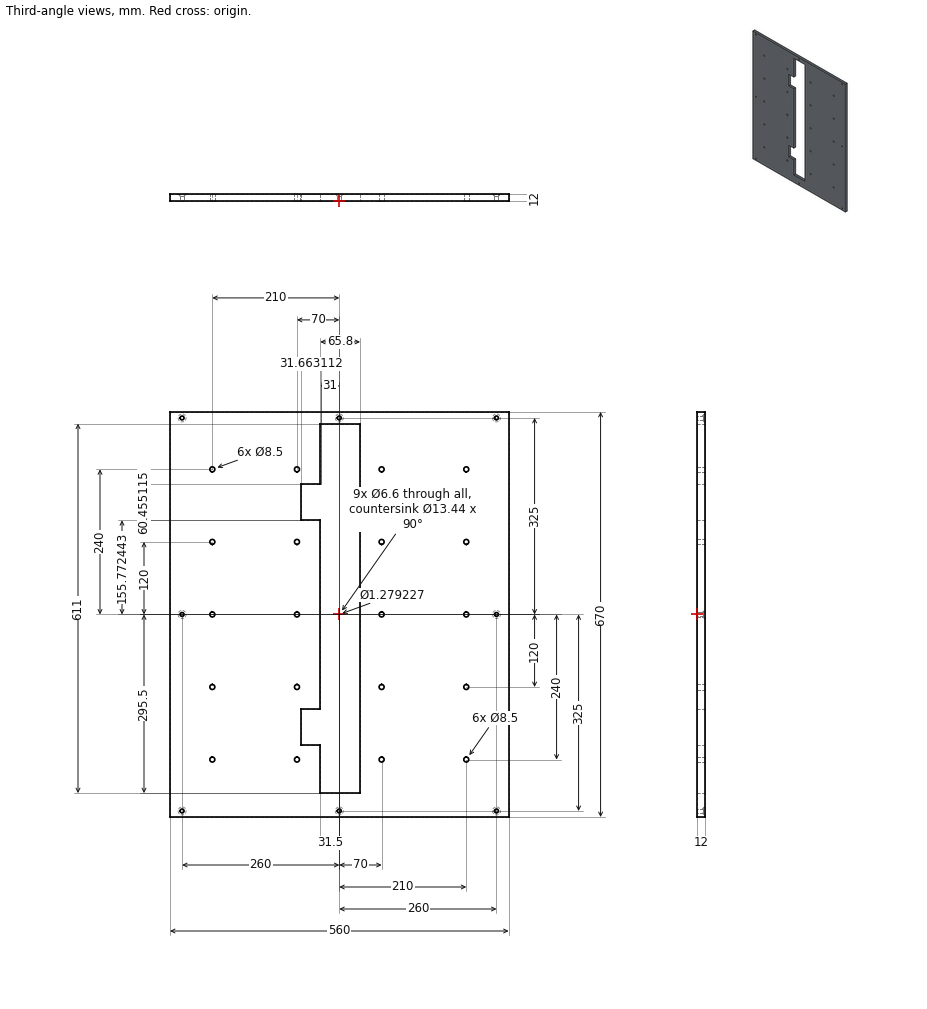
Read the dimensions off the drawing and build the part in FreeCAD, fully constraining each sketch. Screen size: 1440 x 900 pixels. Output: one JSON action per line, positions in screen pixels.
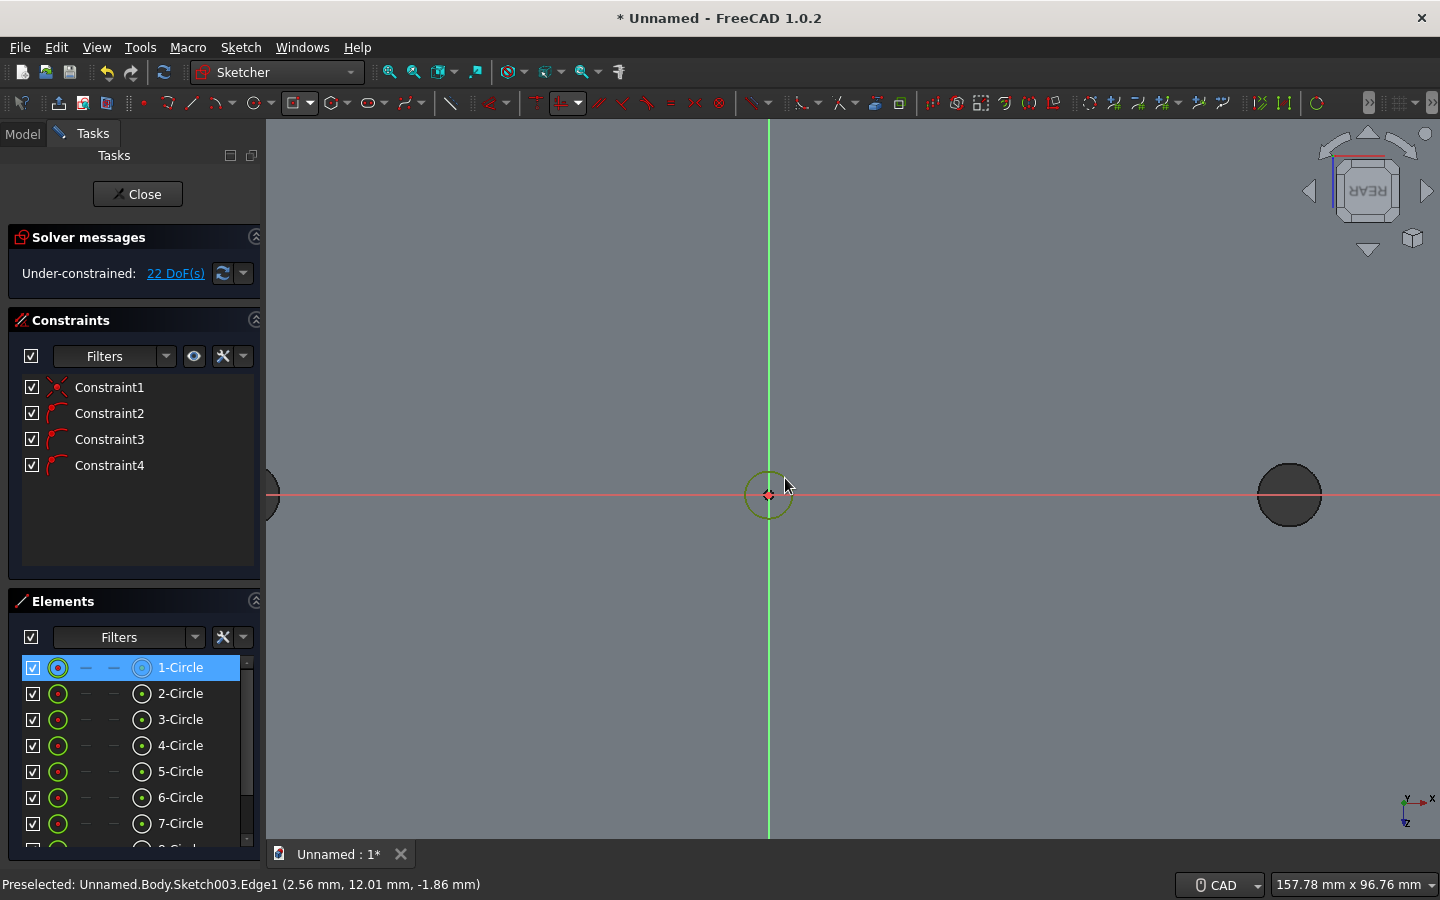
{"action": "scroll", "coordinate": [786, 477], "scroll_direction": "down", "scroll_amount": 12}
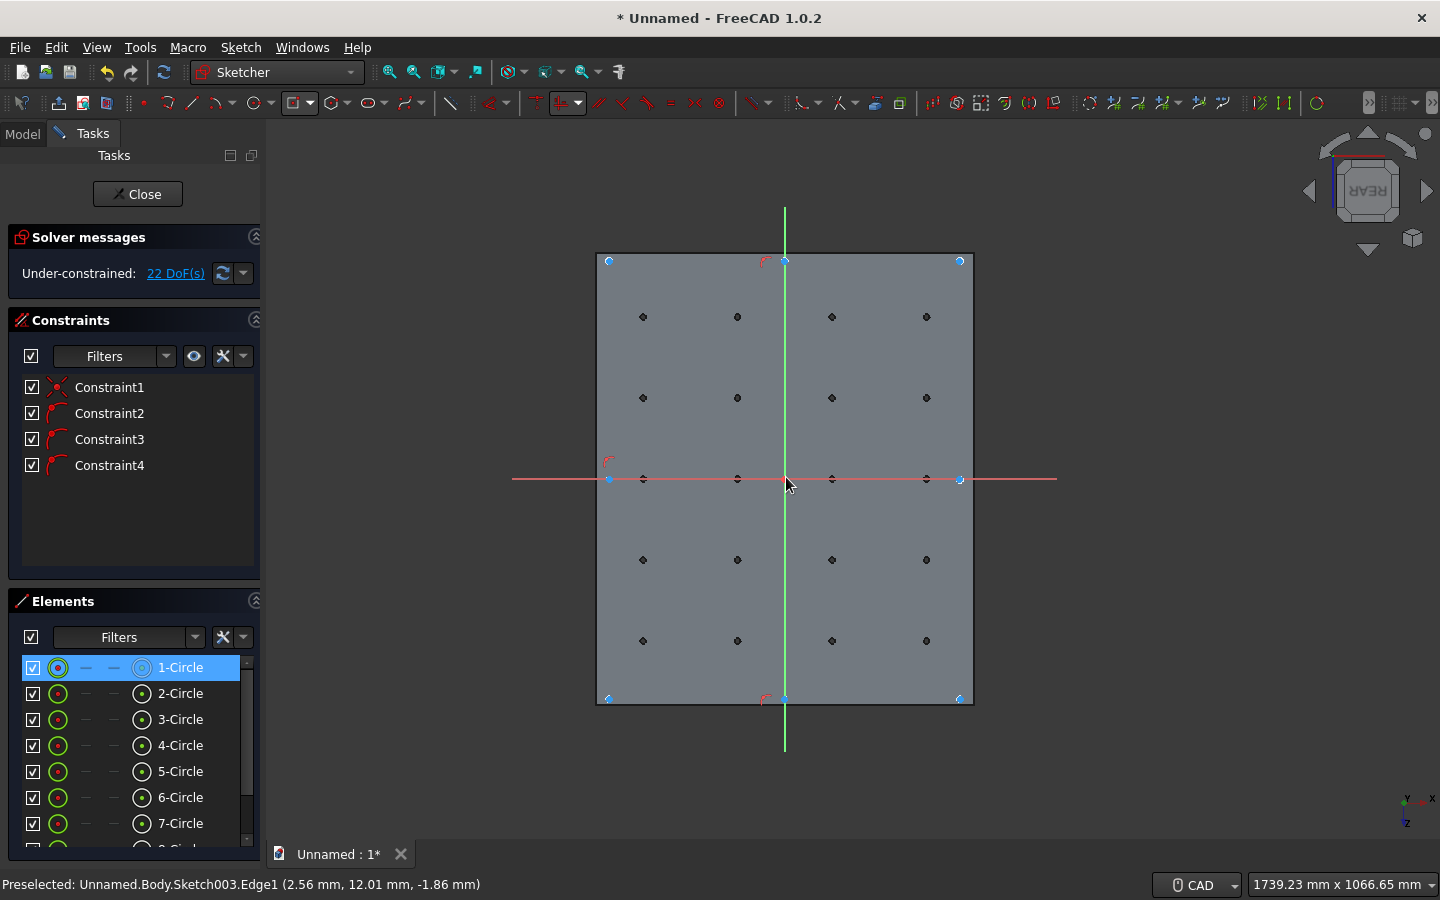
{"action": "scroll", "coordinate": [962, 478], "scroll_direction": "up", "scroll_amount": 12}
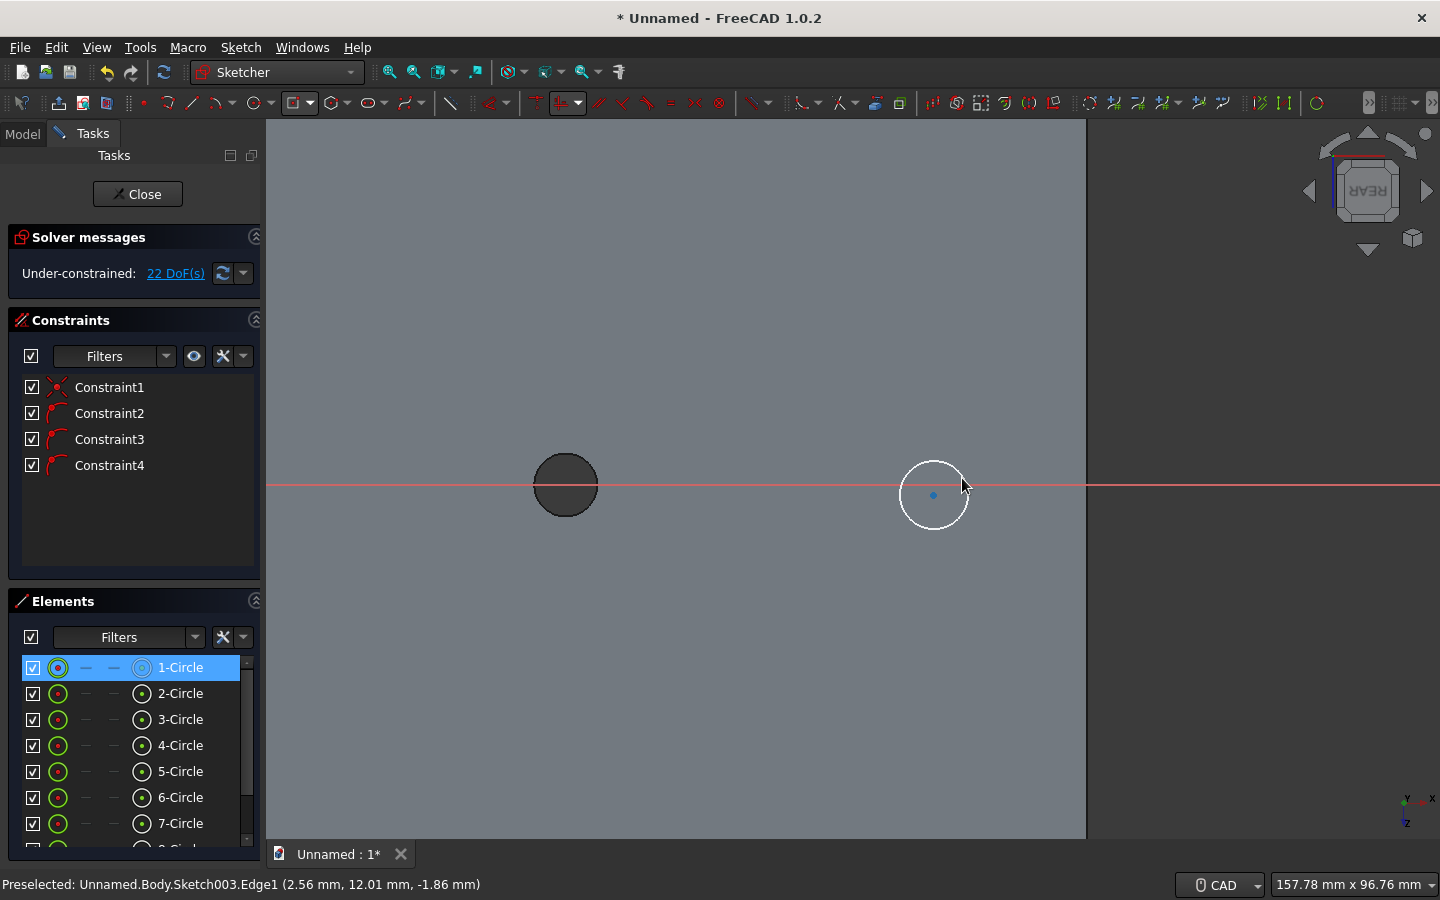
{"action": "left_click", "coordinate": [958, 471]}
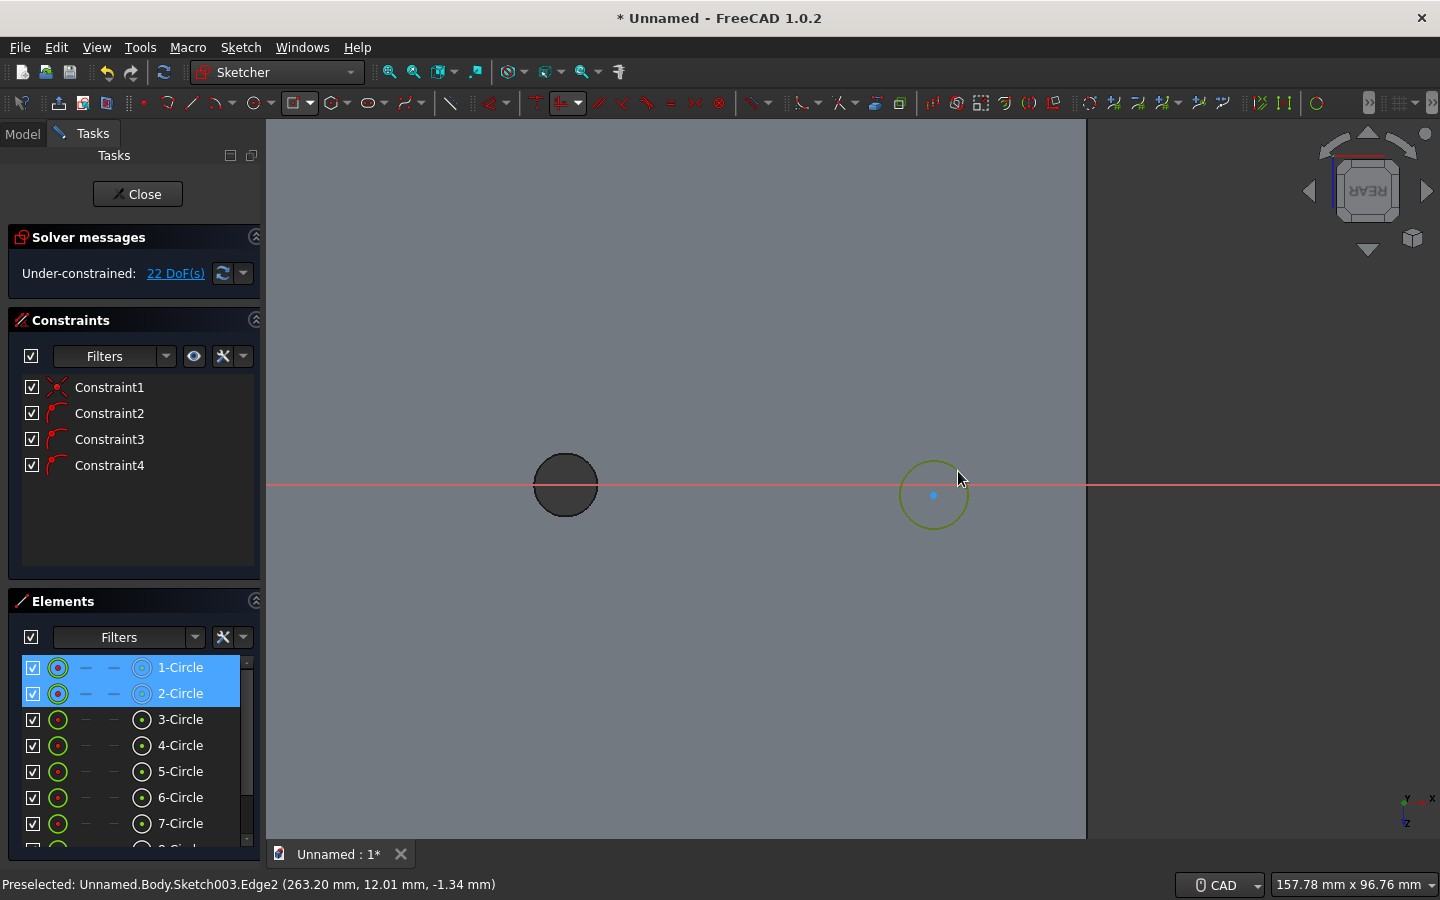
{"action": "scroll", "coordinate": [962, 478], "scroll_direction": "down", "scroll_amount": 12}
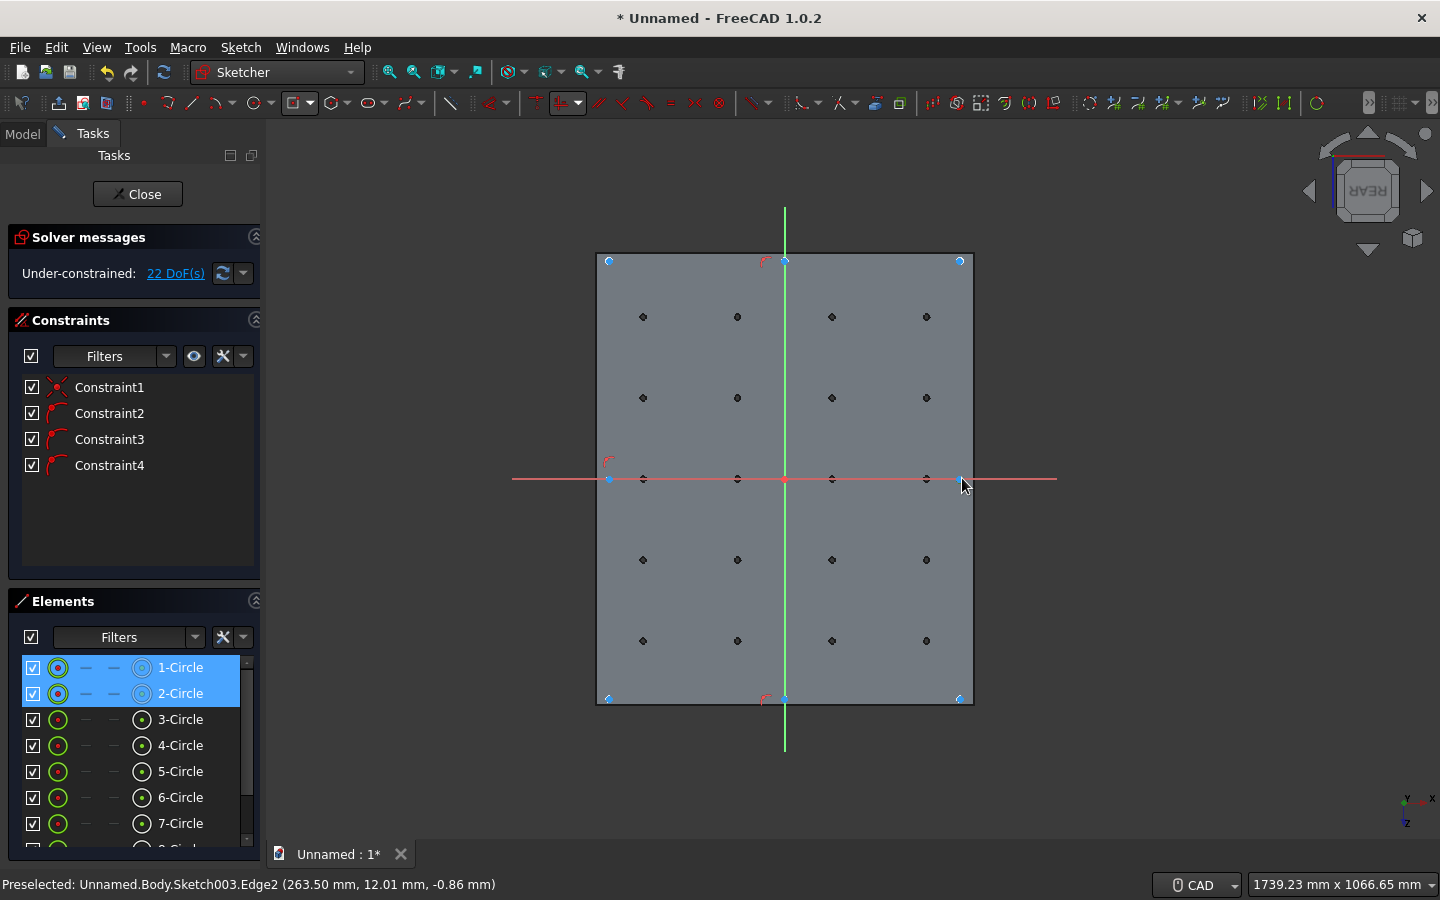
{"action": "scroll", "coordinate": [787, 259], "scroll_direction": "up", "scroll_amount": 10}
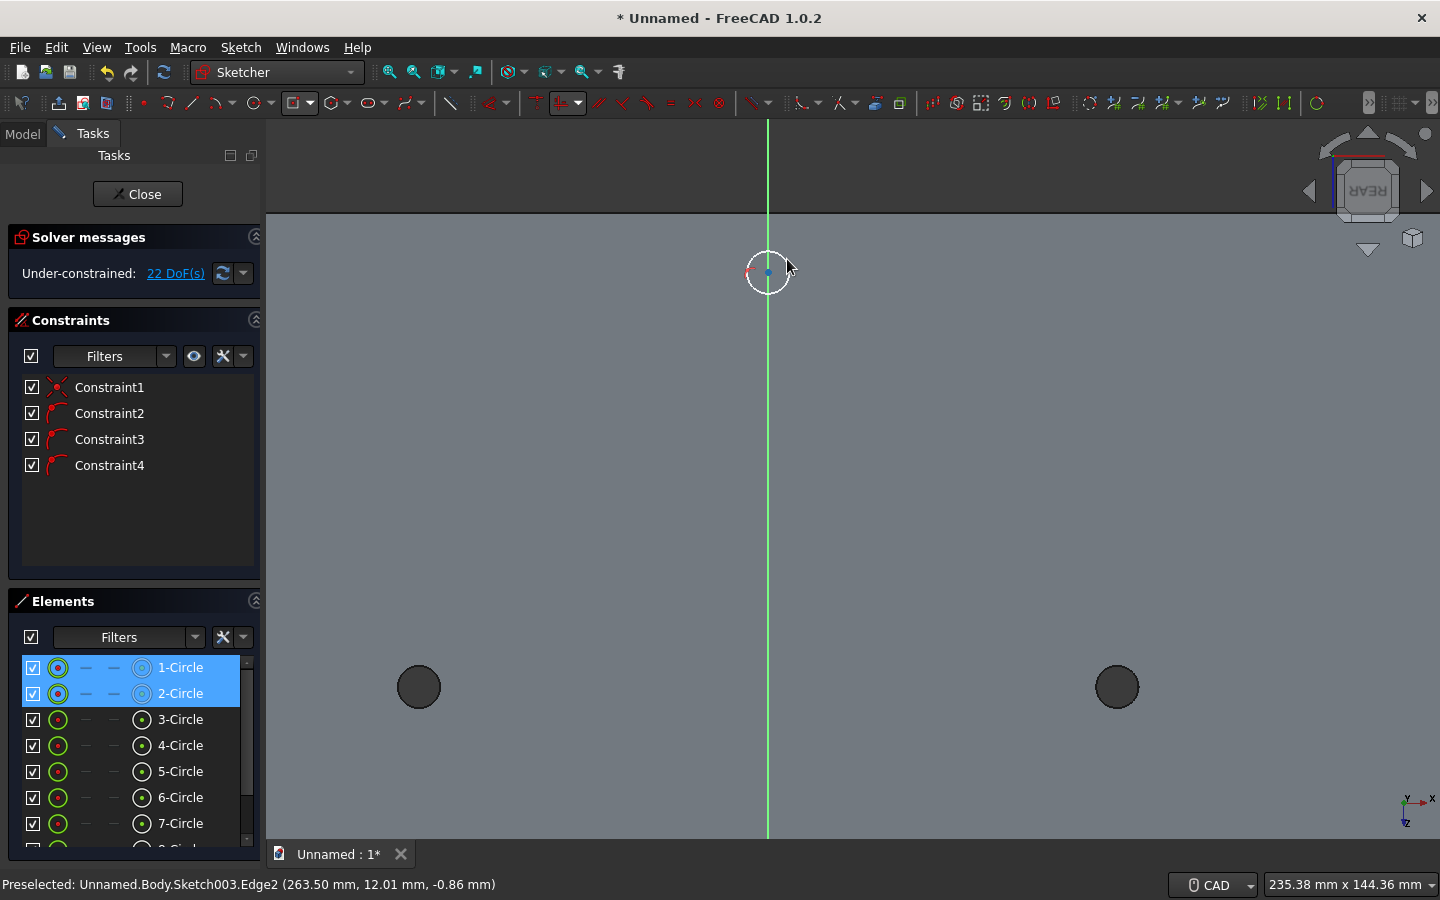
{"action": "left_click", "coordinate": [783, 258]}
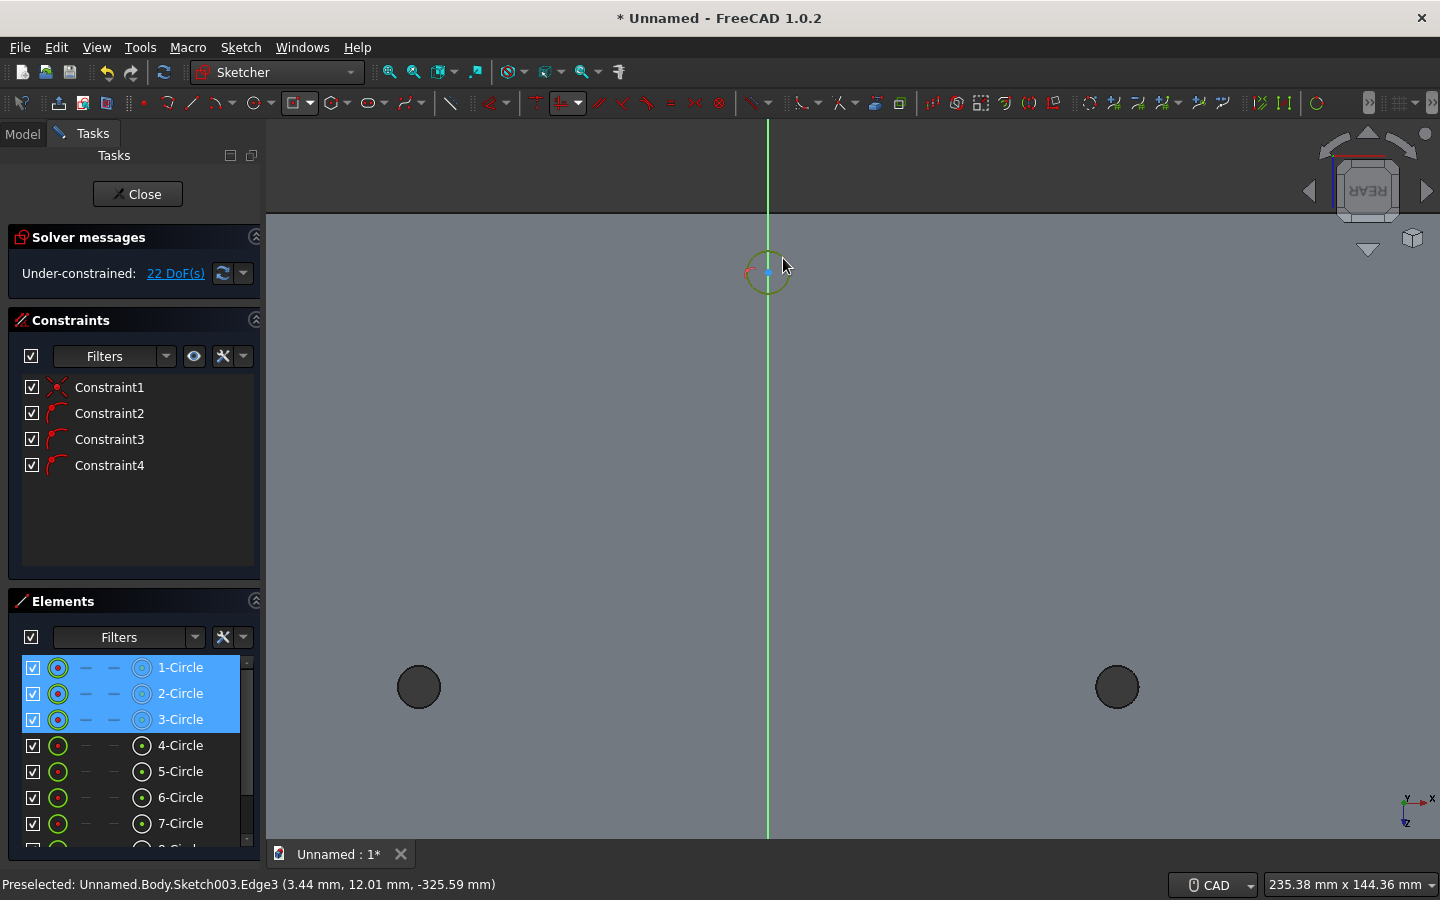
{"action": "scroll", "coordinate": [787, 259], "scroll_direction": "down", "scroll_amount": 10}